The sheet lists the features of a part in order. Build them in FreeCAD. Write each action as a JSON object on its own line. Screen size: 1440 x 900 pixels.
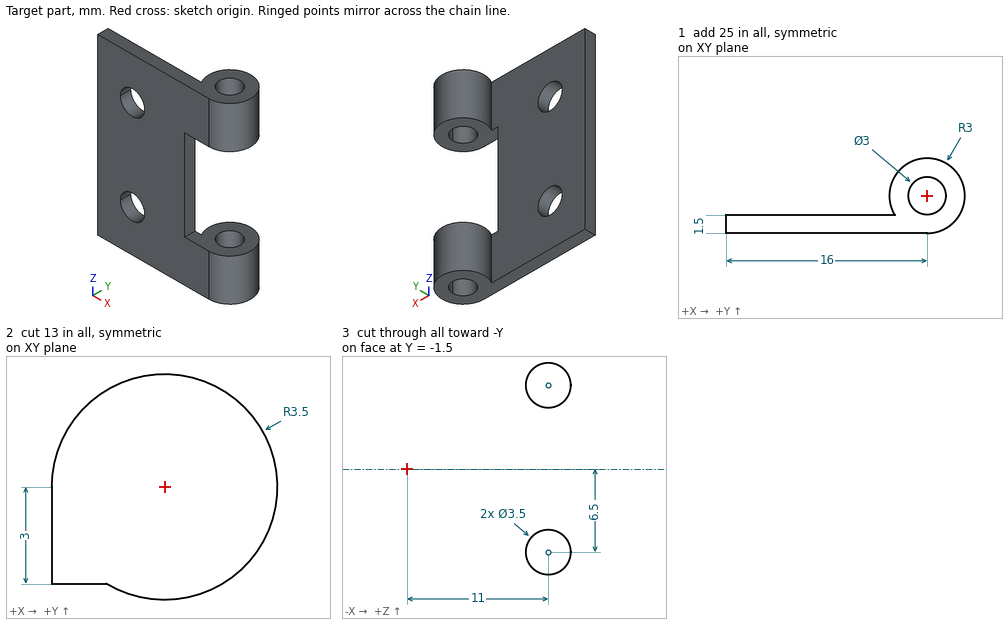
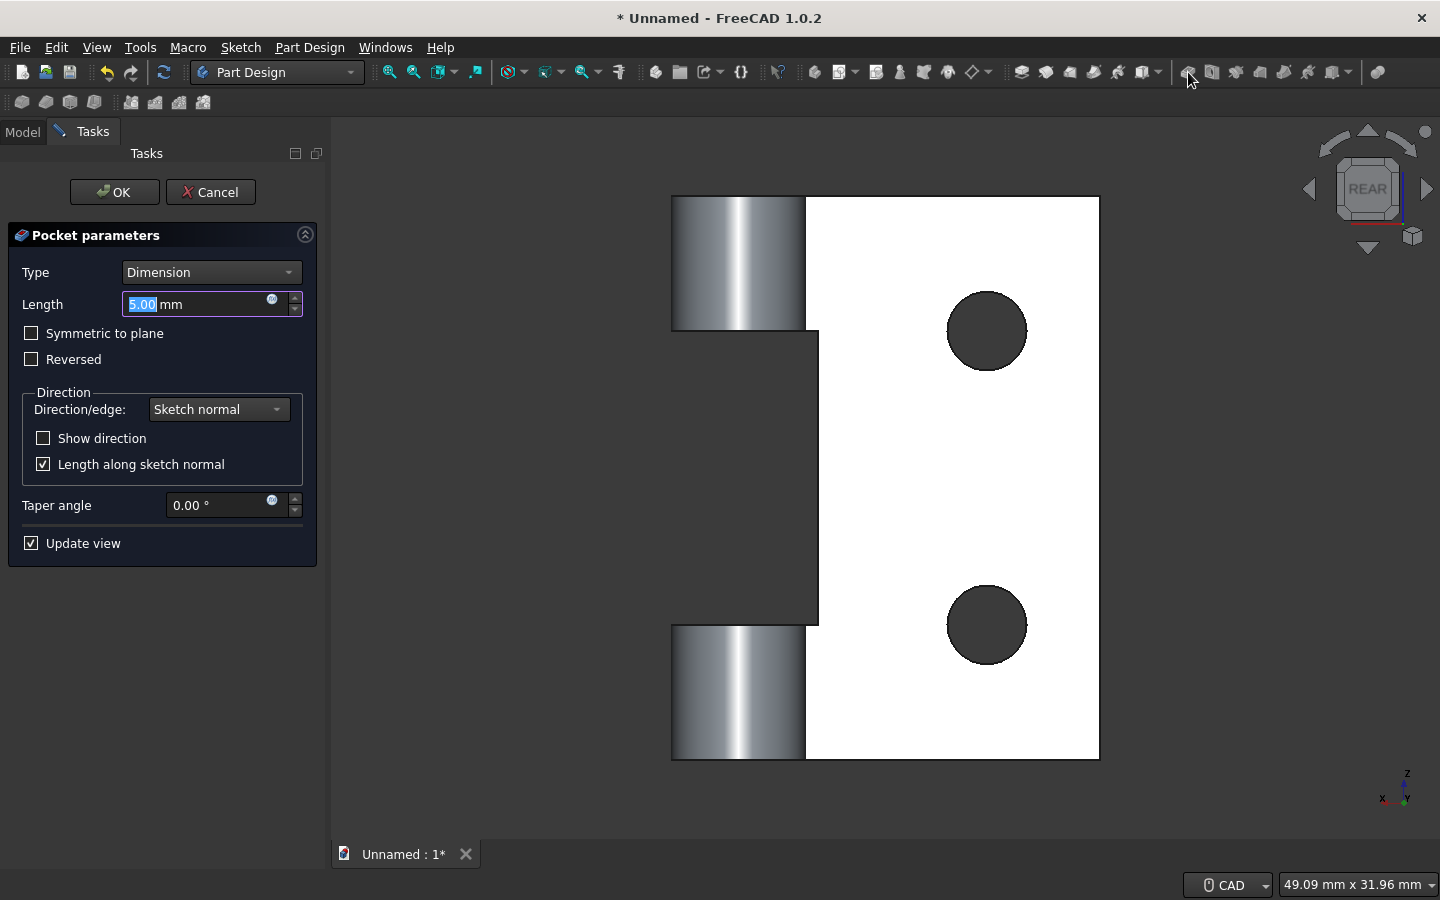
{"action": "left_click", "coordinate": [212, 272]}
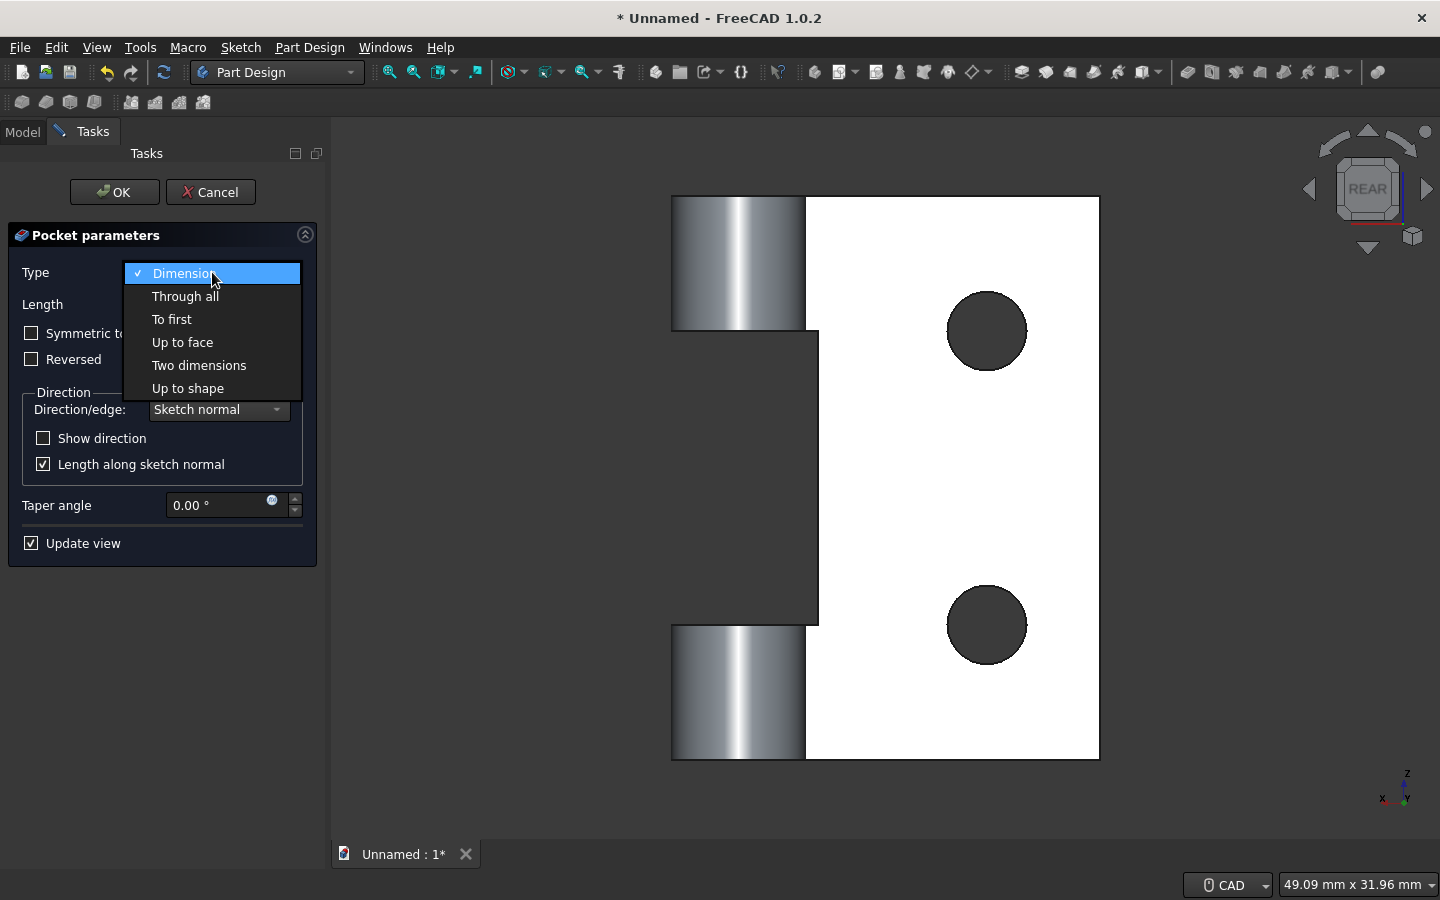
{"action": "left_click", "coordinate": [212, 296]}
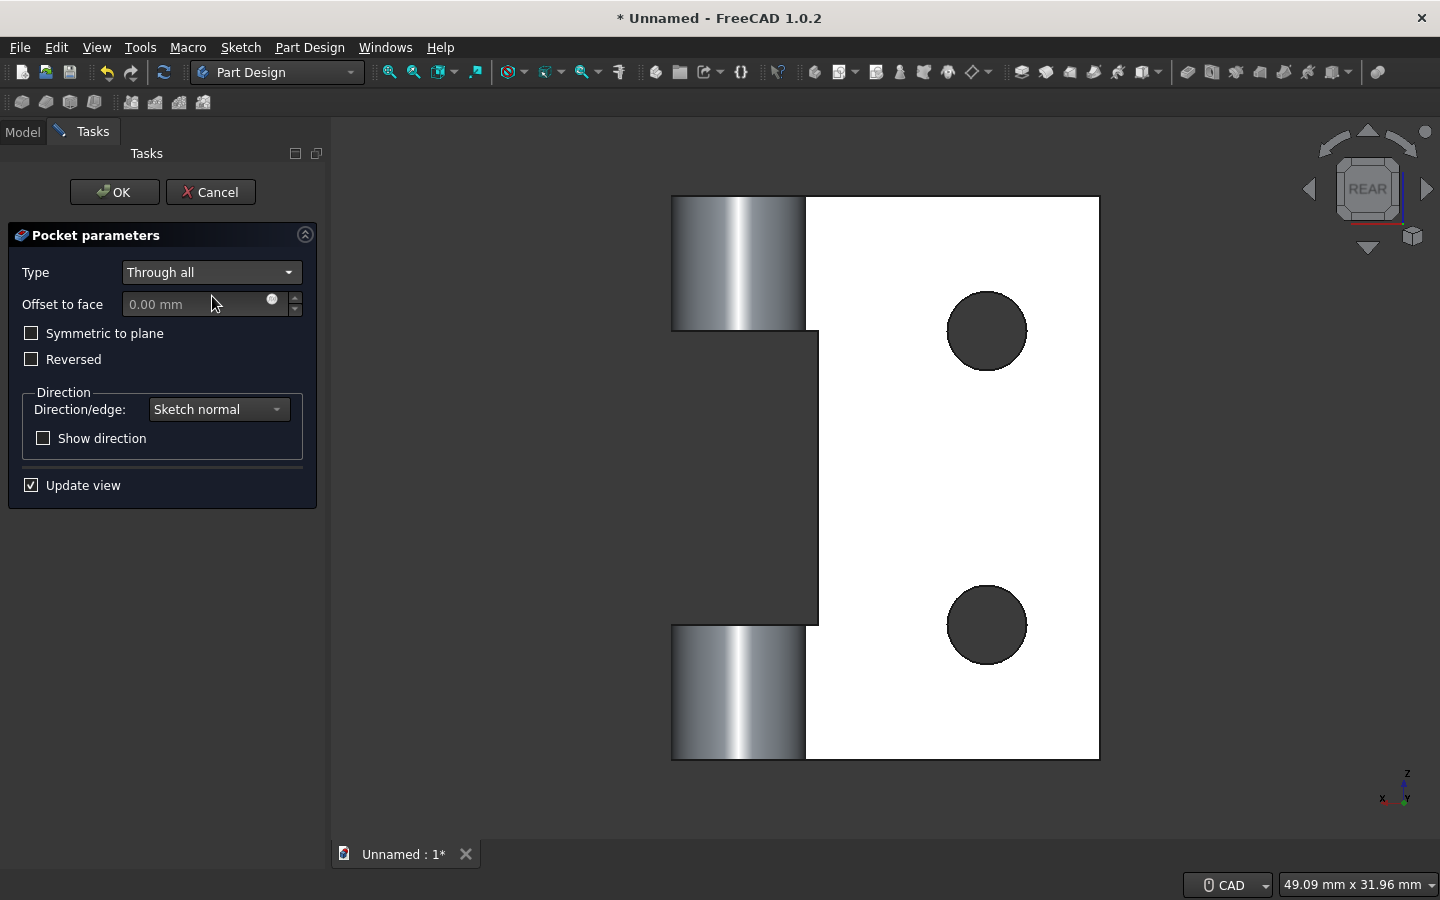
{"action": "left_click", "coordinate": [115, 192]}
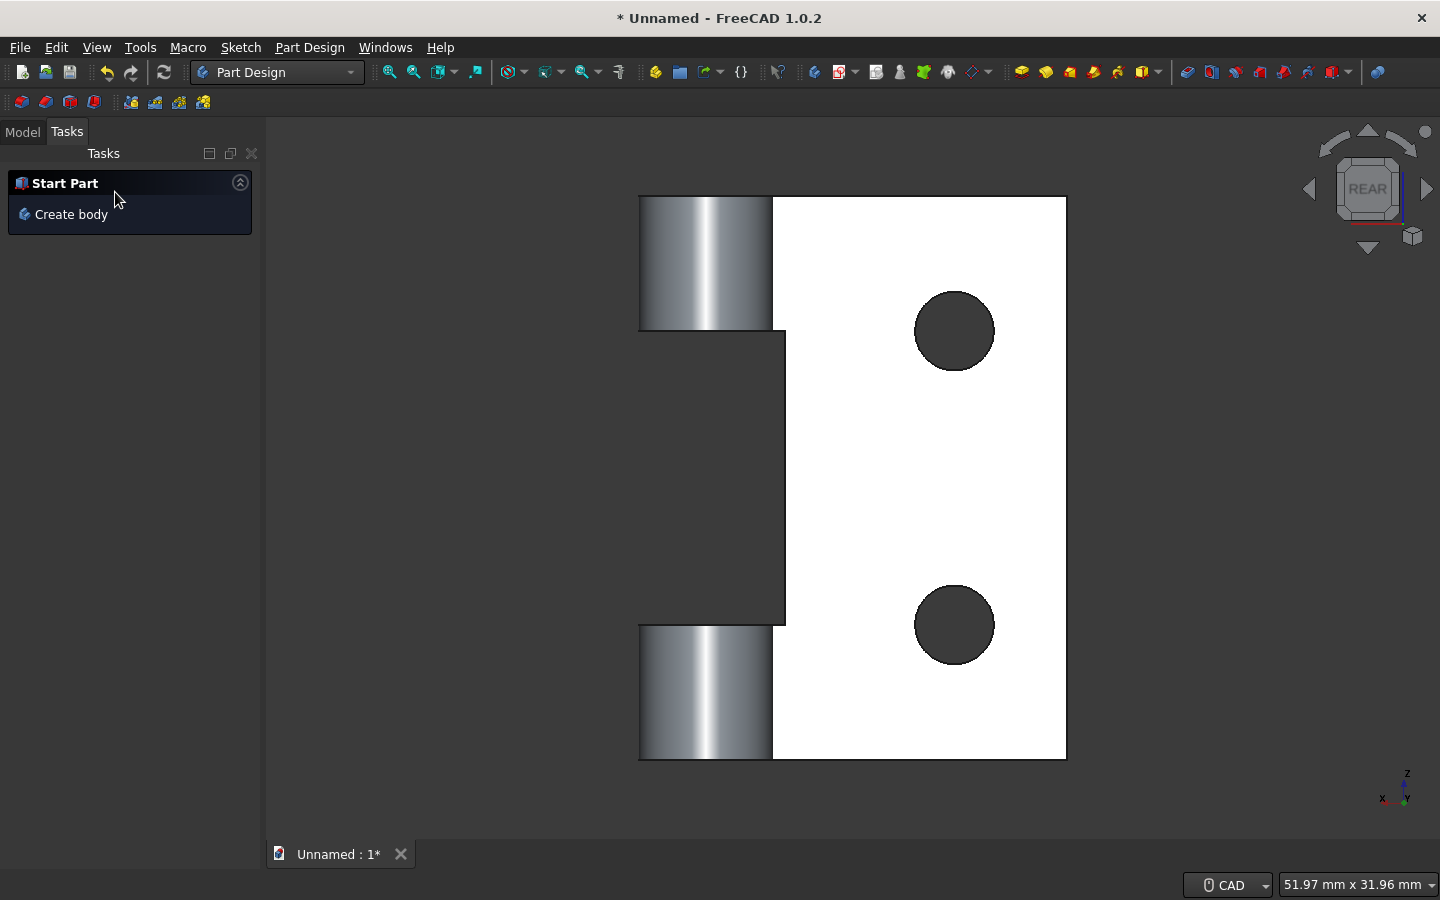
{"action": "key", "text": "0"}